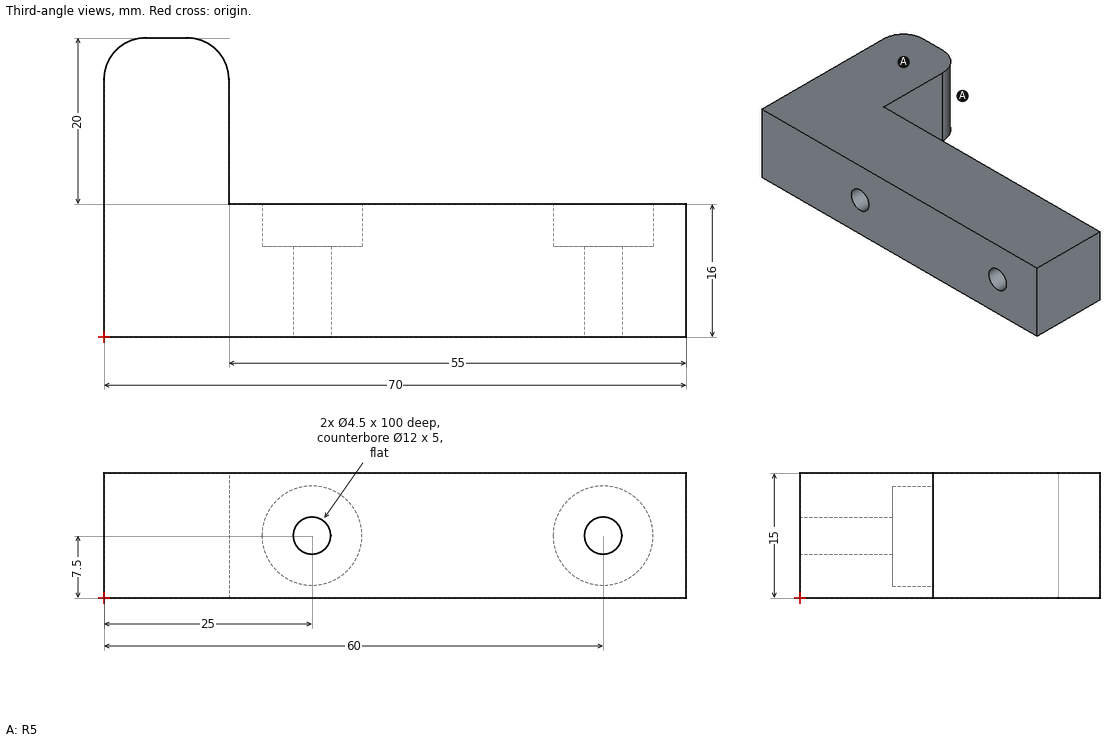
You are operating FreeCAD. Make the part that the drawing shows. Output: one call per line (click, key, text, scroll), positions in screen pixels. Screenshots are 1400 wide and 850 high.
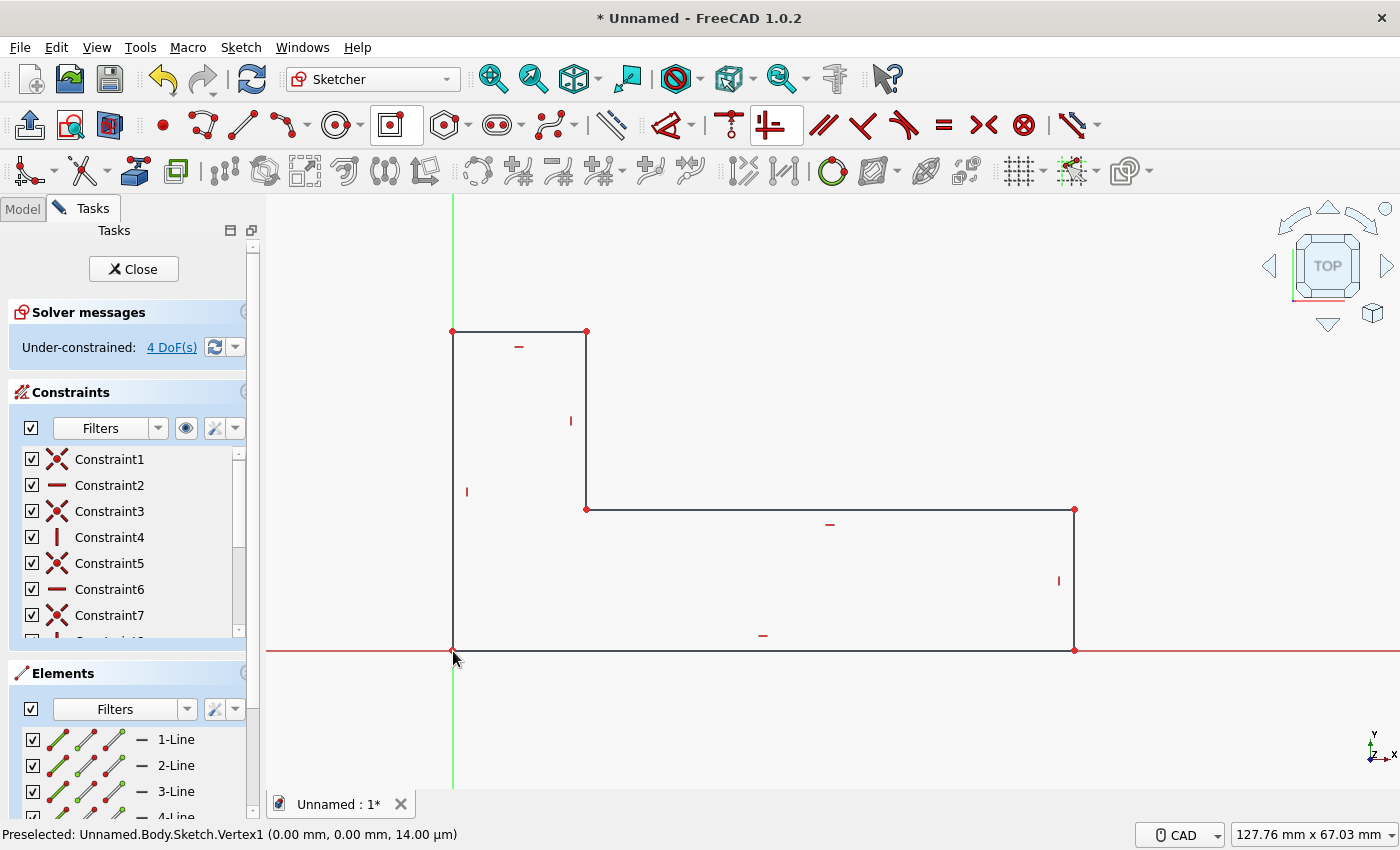
click(639, 651)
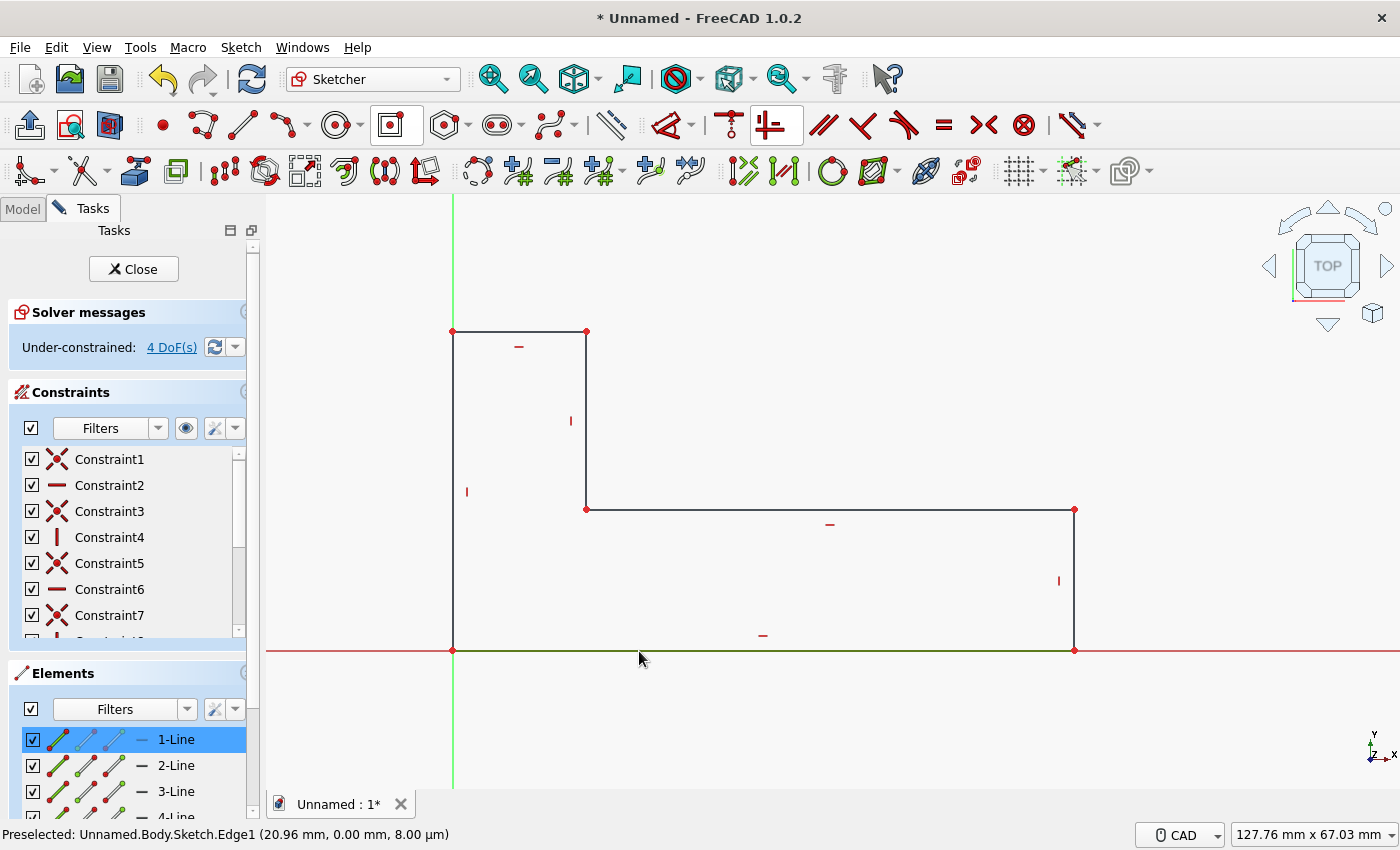
click(694, 126)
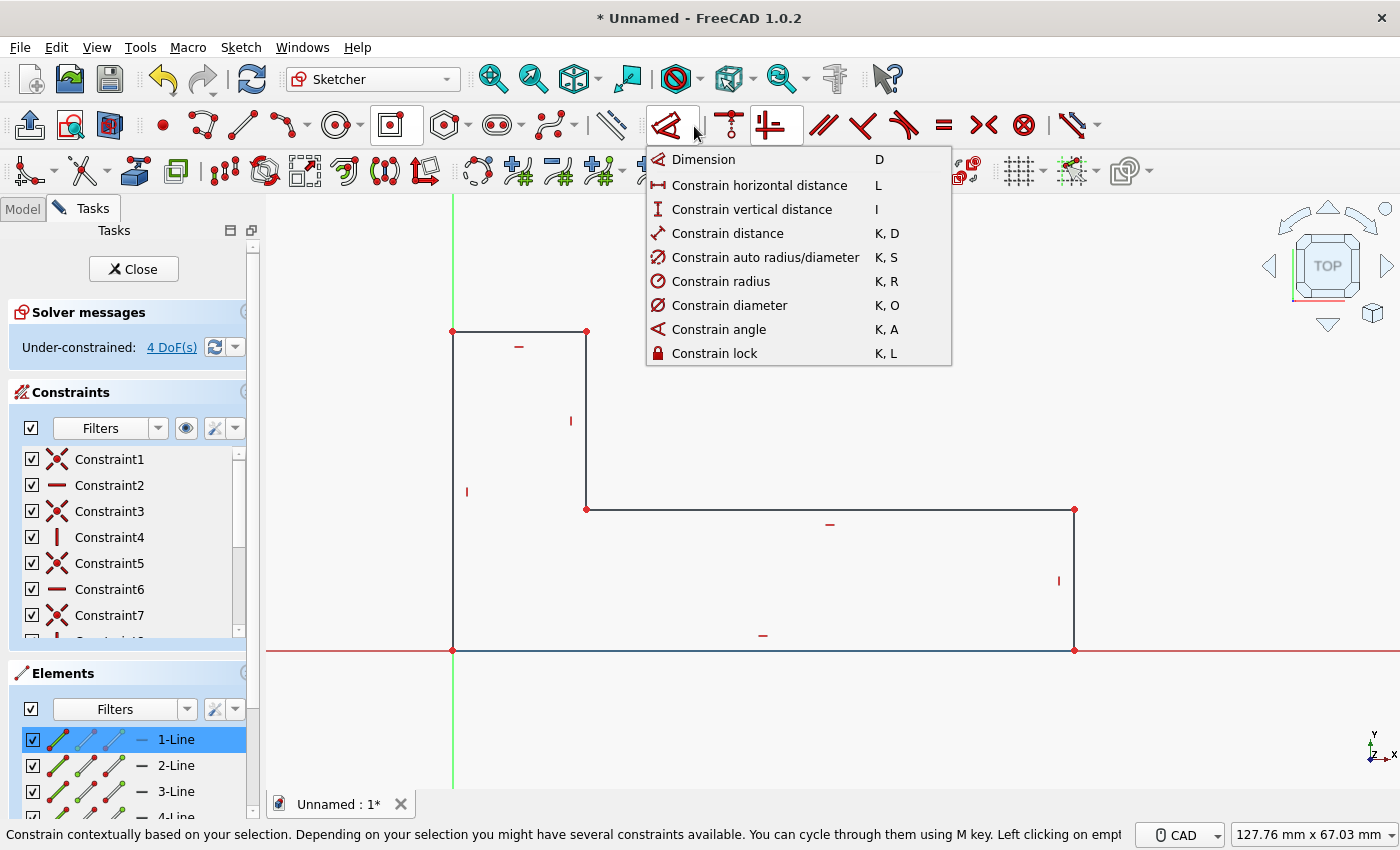
click(799, 185)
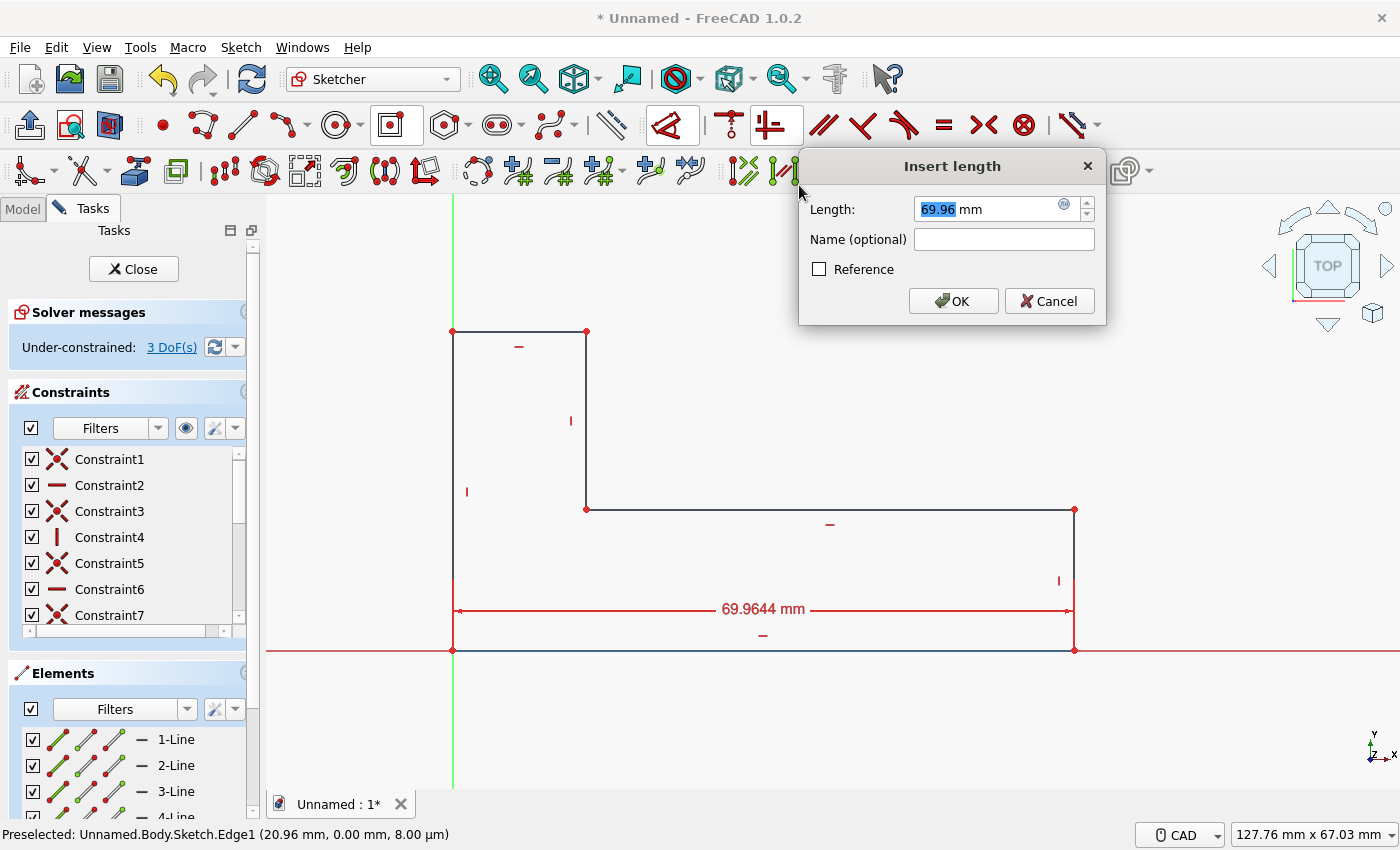
text(70)
key(Return)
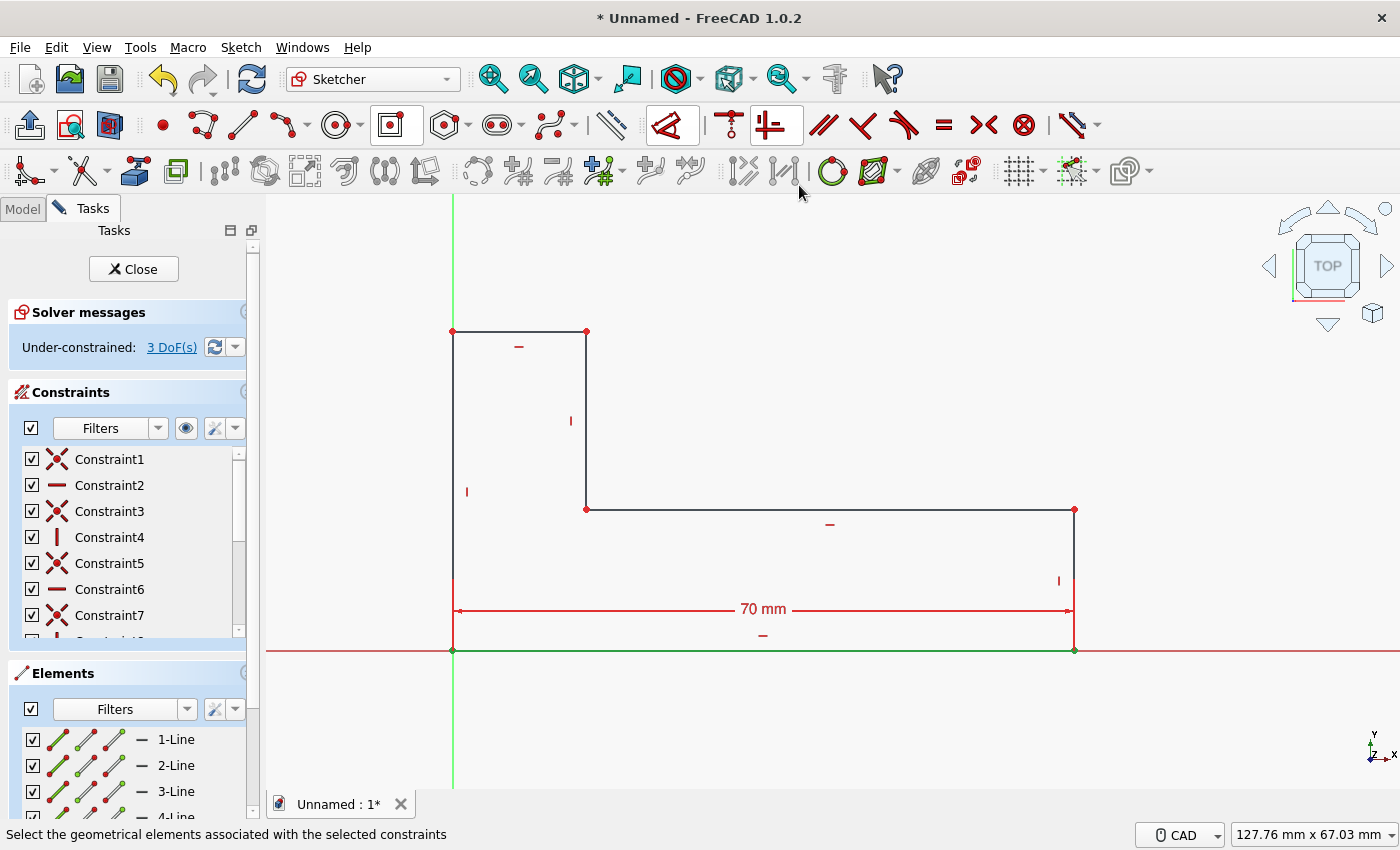
click(1074, 609)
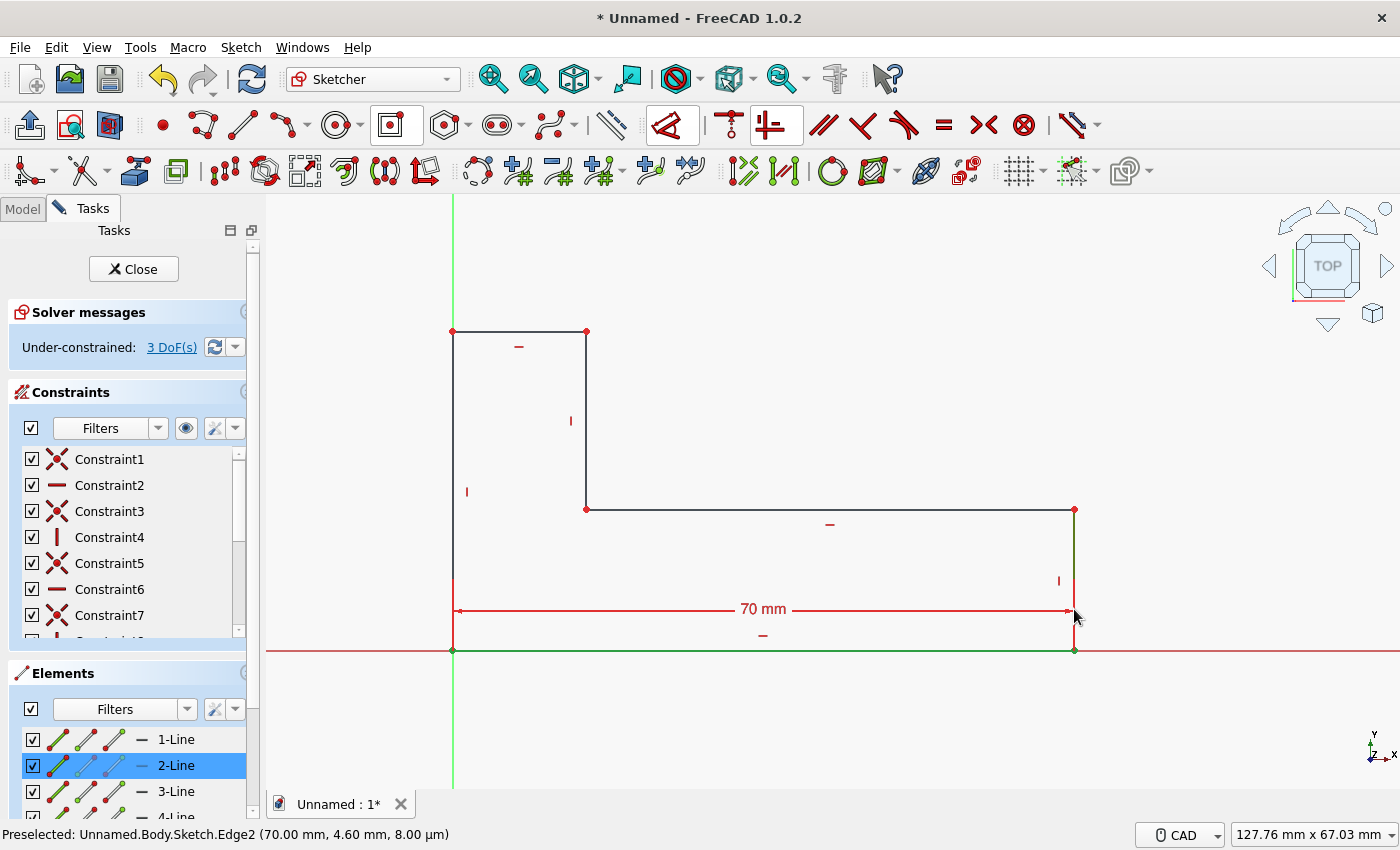
key(i)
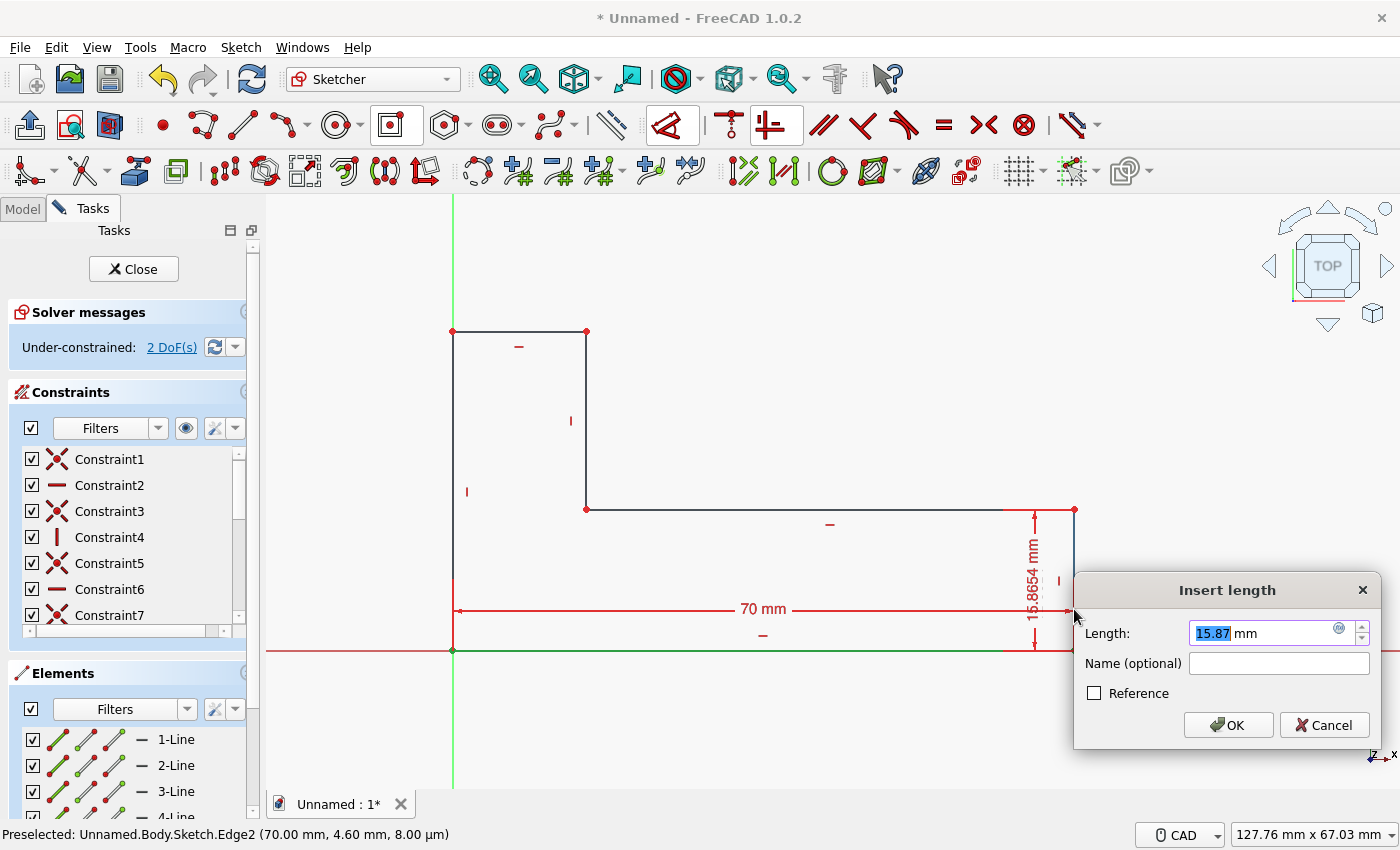
text(16)
key(Return)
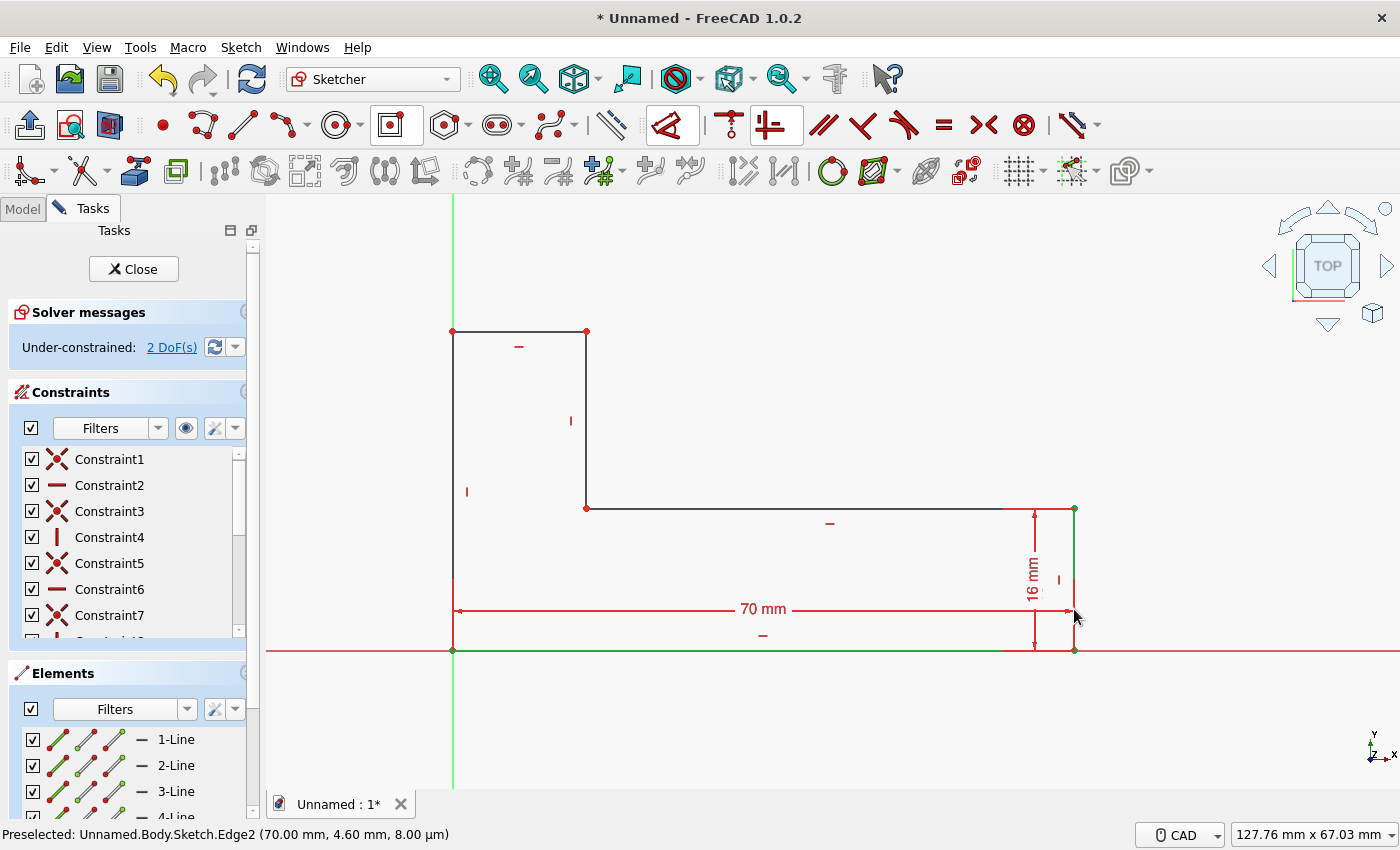
click(928, 509)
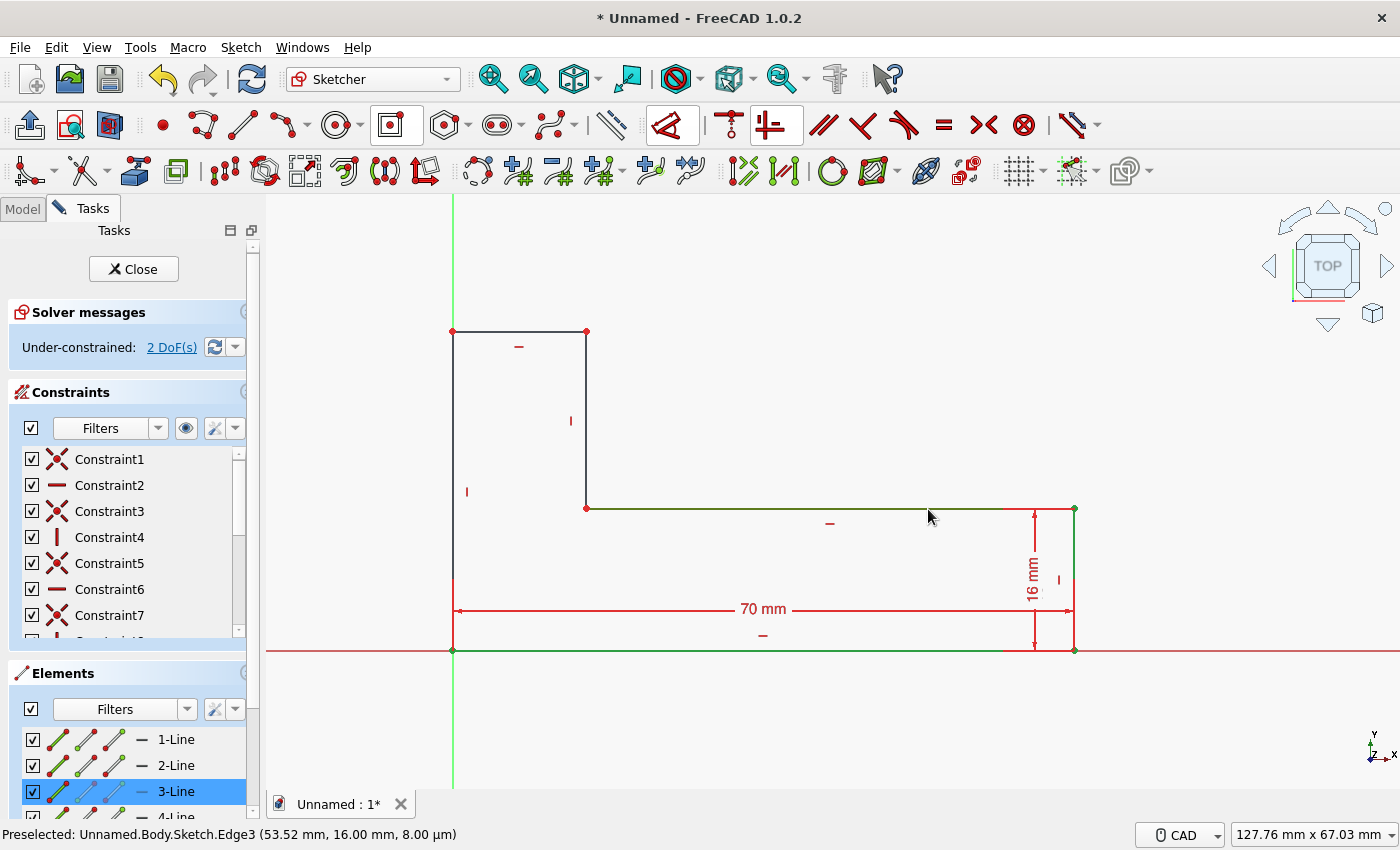
click(694, 126)